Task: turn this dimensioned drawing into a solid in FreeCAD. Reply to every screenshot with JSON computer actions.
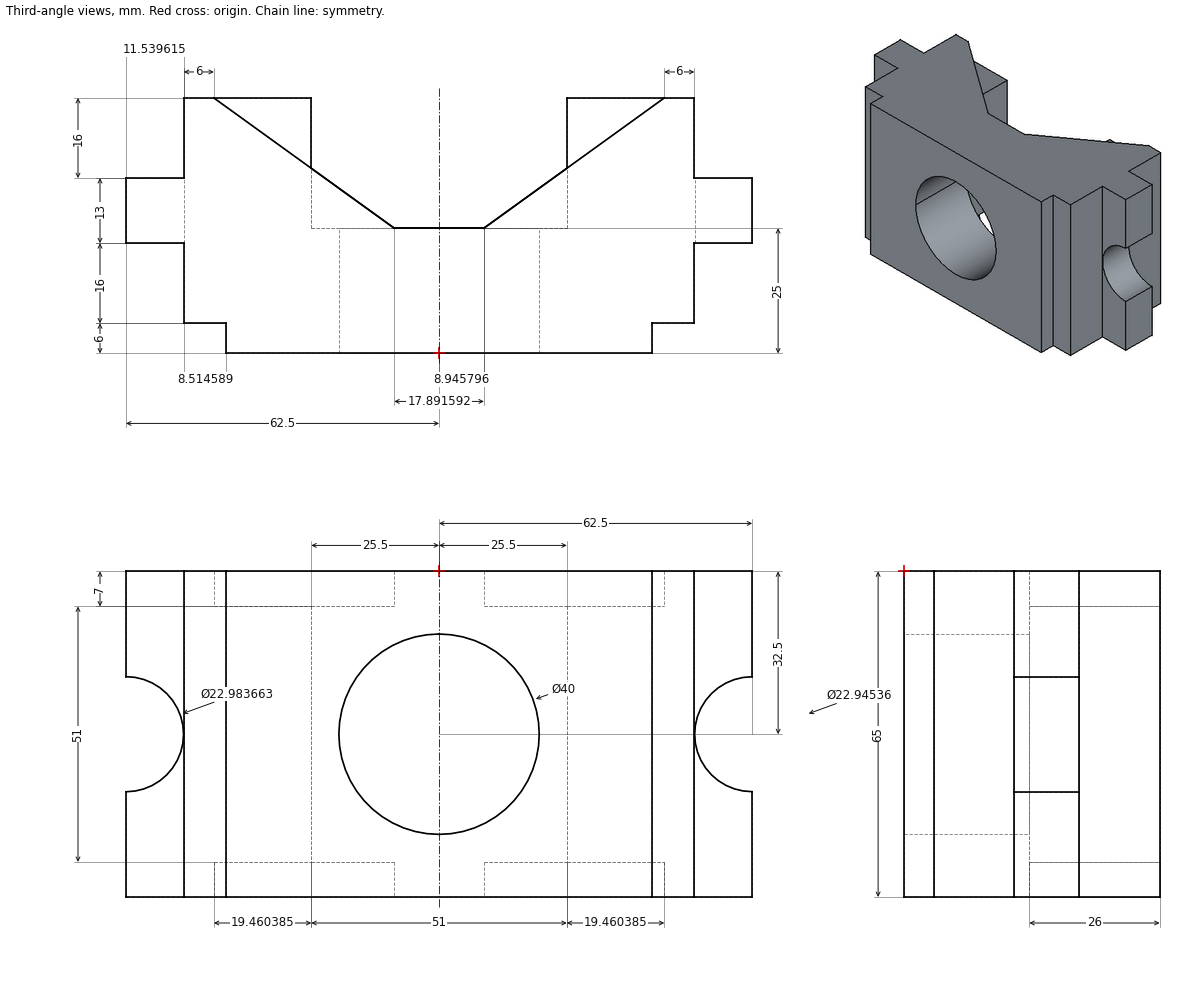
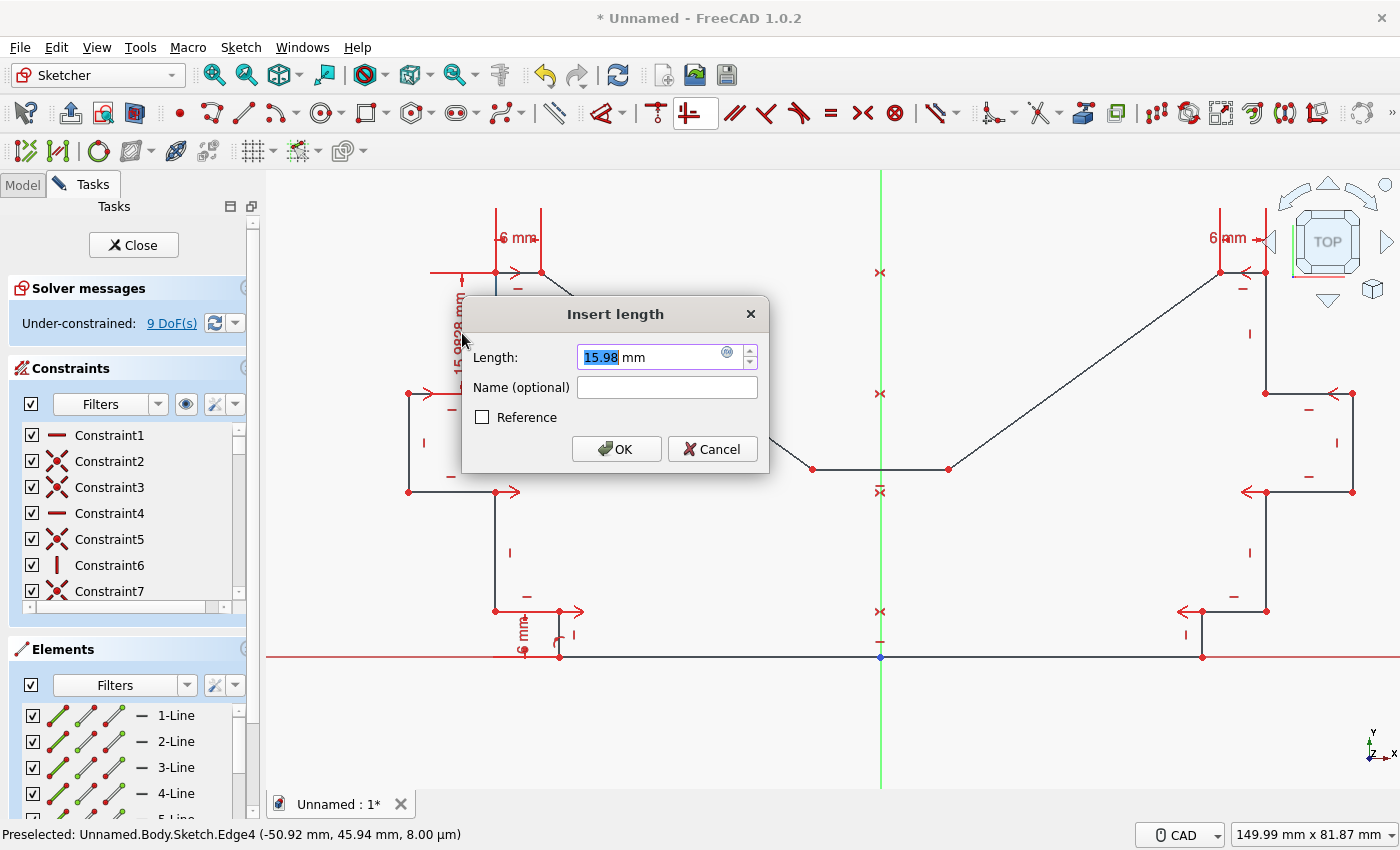
{"action": "type", "text": "16"}
{"action": "key", "text": "Return"}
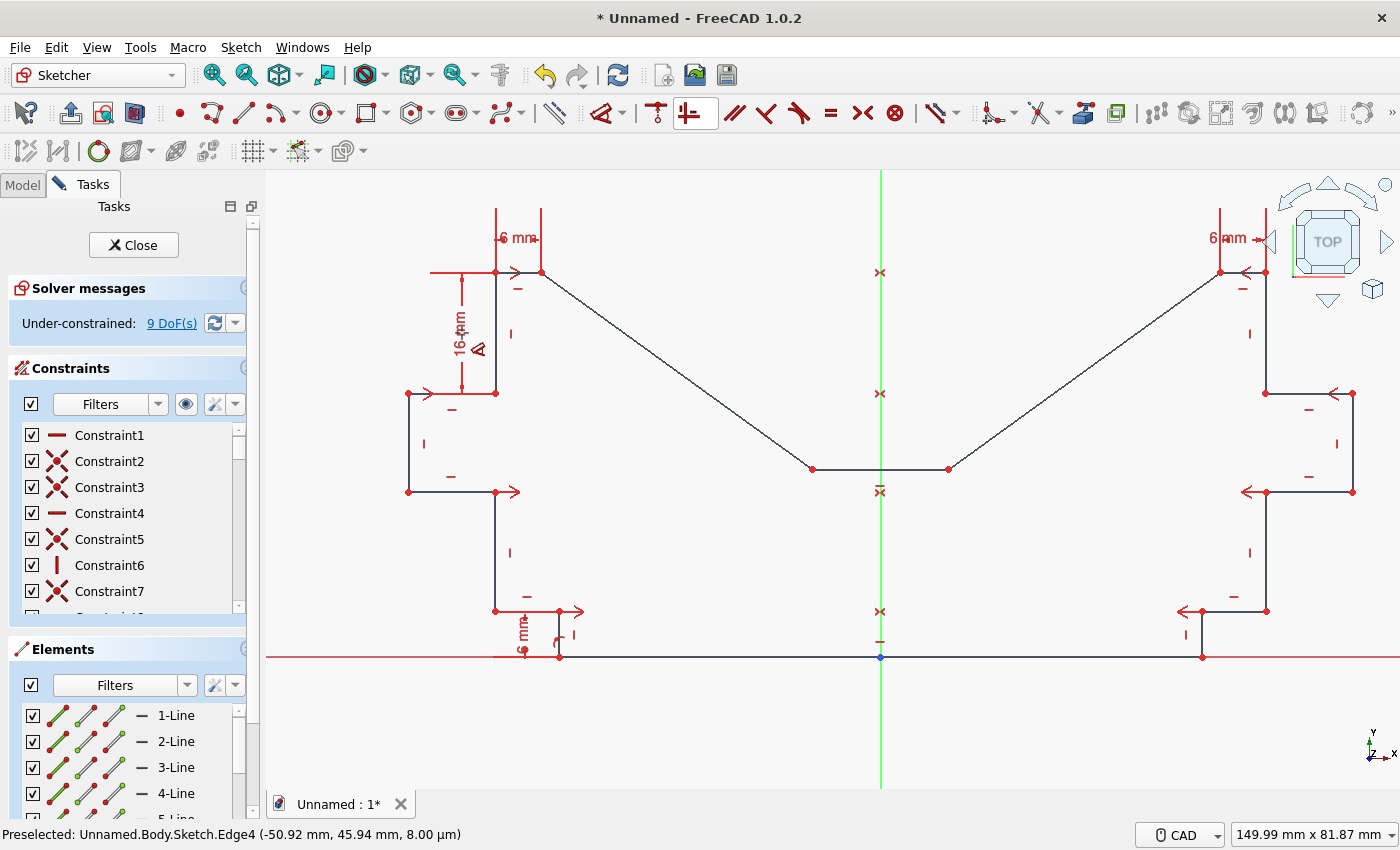
{"action": "left_click", "coordinate": [409, 423]}
{"action": "left_click", "coordinate": [375, 443]}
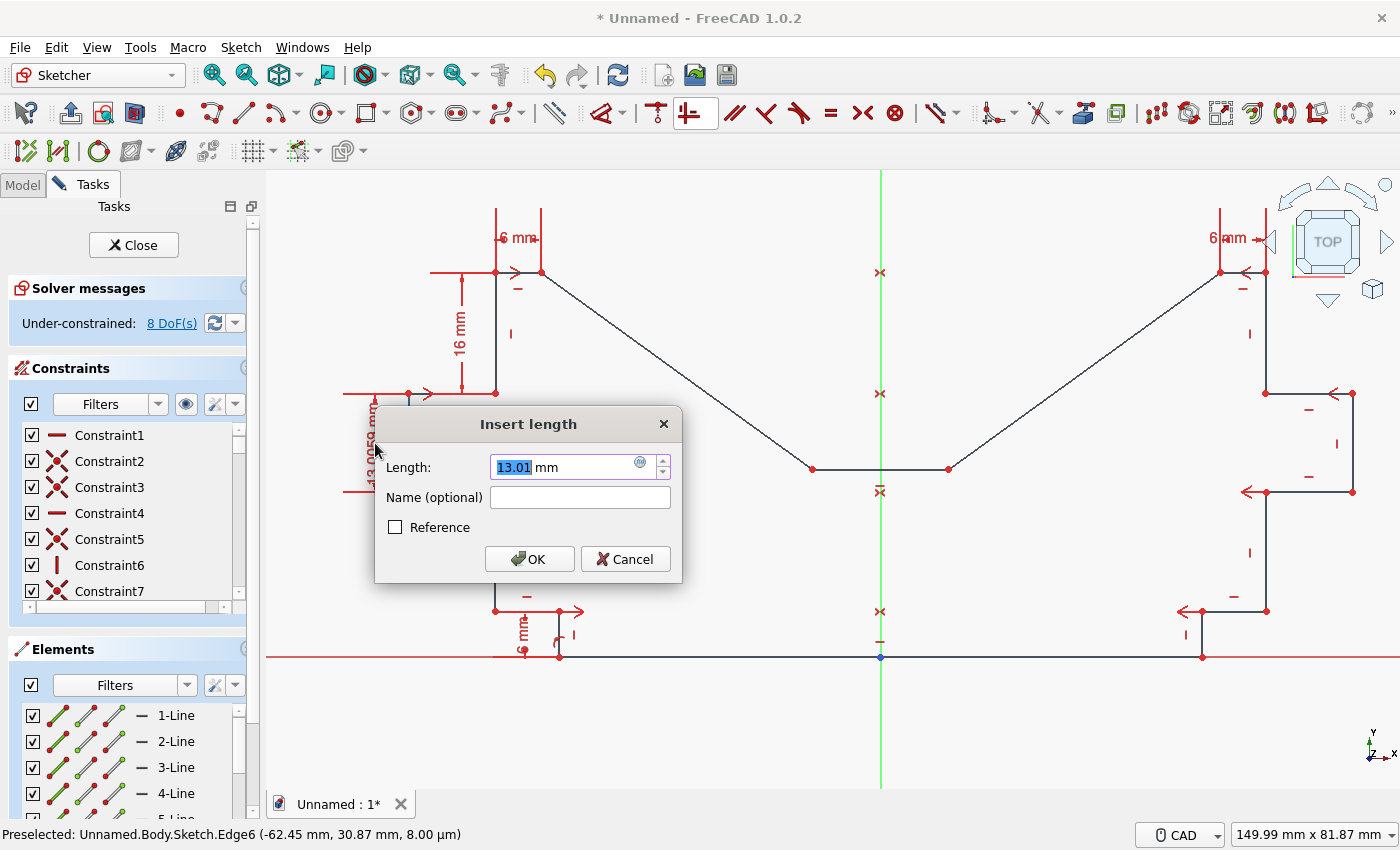
{"action": "type", "text": "13"}
{"action": "key", "text": "Return"}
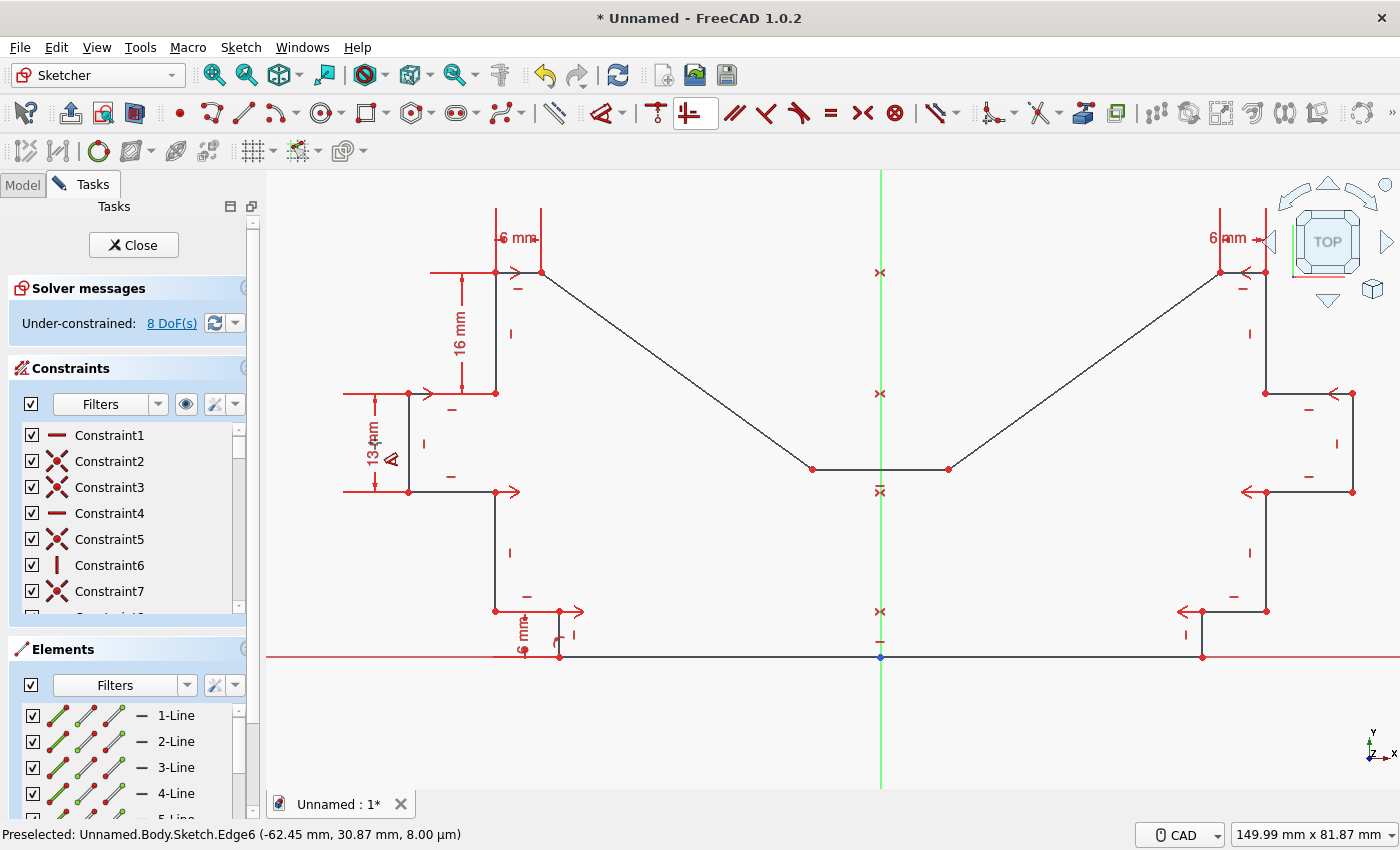
{"action": "left_click", "coordinate": [495, 528]}
{"action": "left_click", "coordinate": [461, 552]}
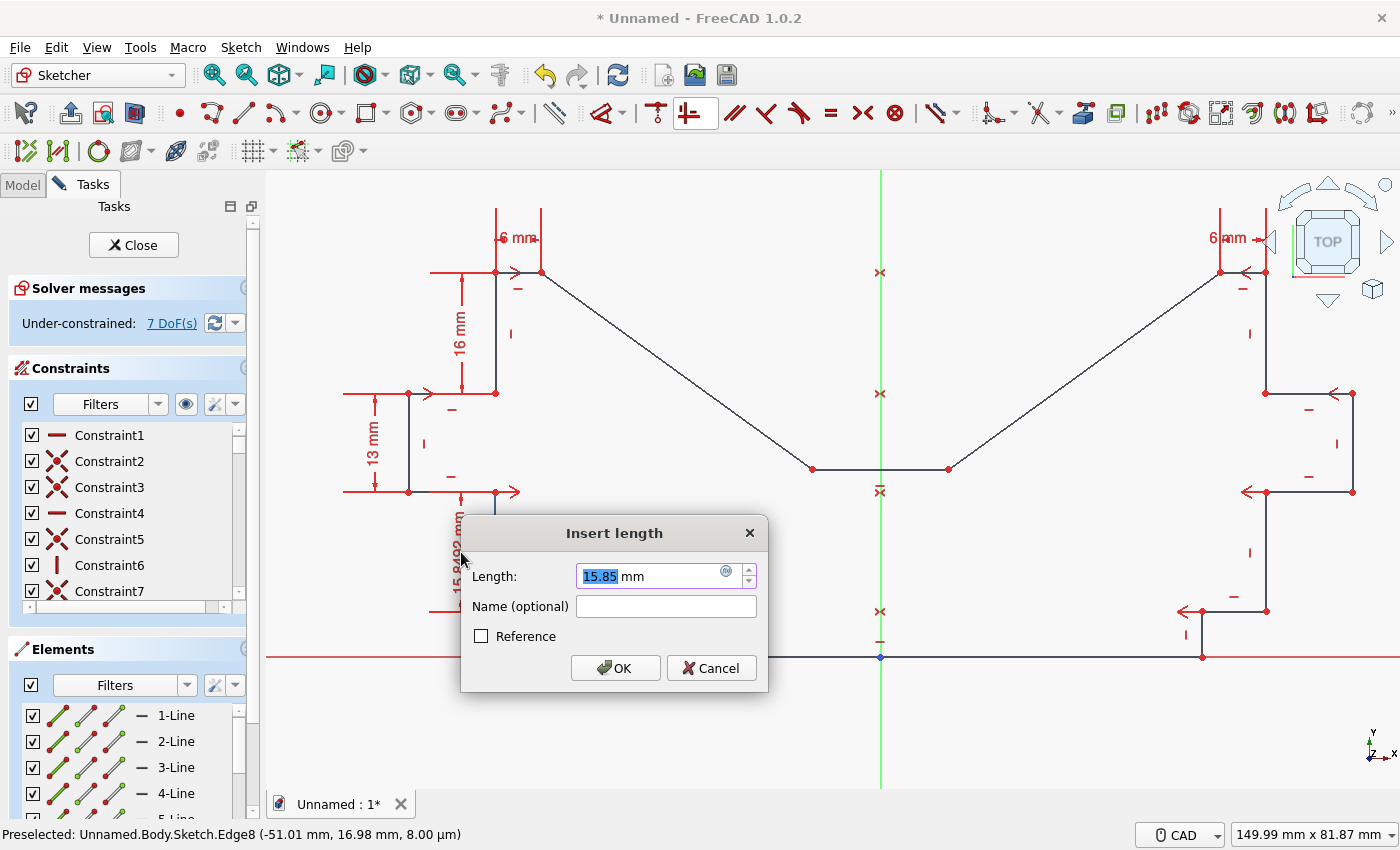
{"action": "type", "text": "16"}
{"action": "key", "text": "Return"}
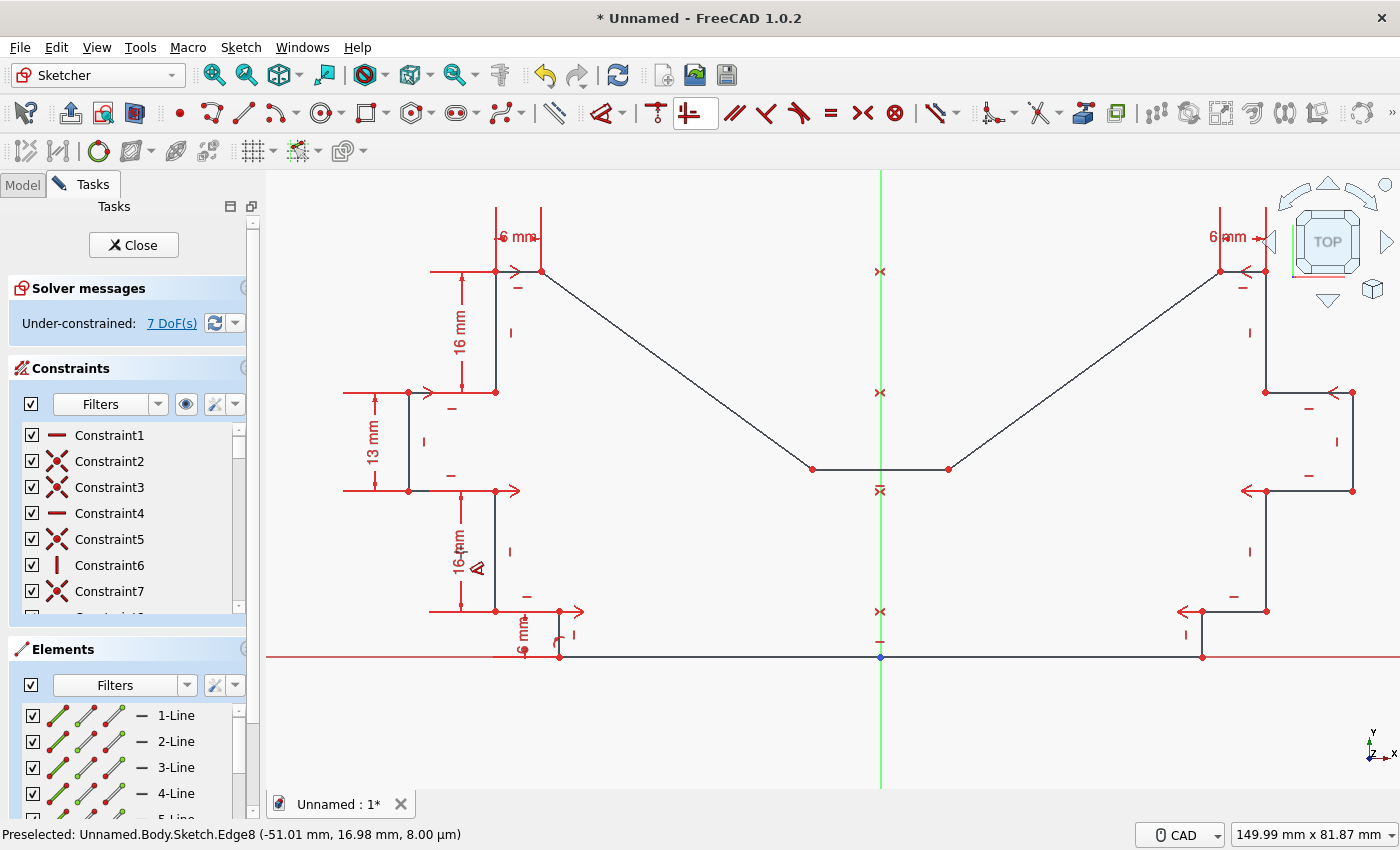
{"action": "left_click", "coordinate": [949, 470]}
{"action": "left_click", "coordinate": [983, 564]}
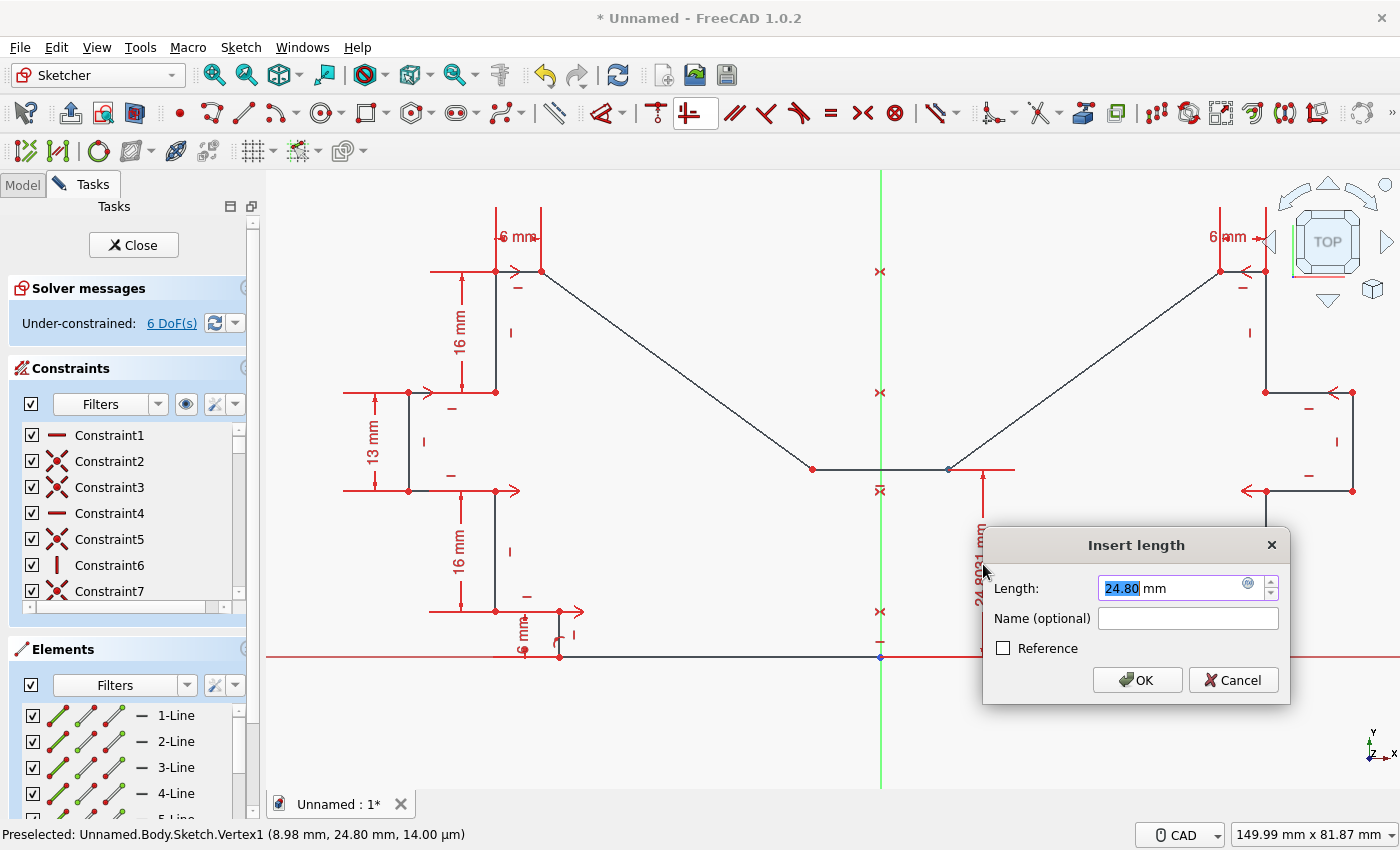
{"action": "type", "text": "25"}
{"action": "key", "text": "Return"}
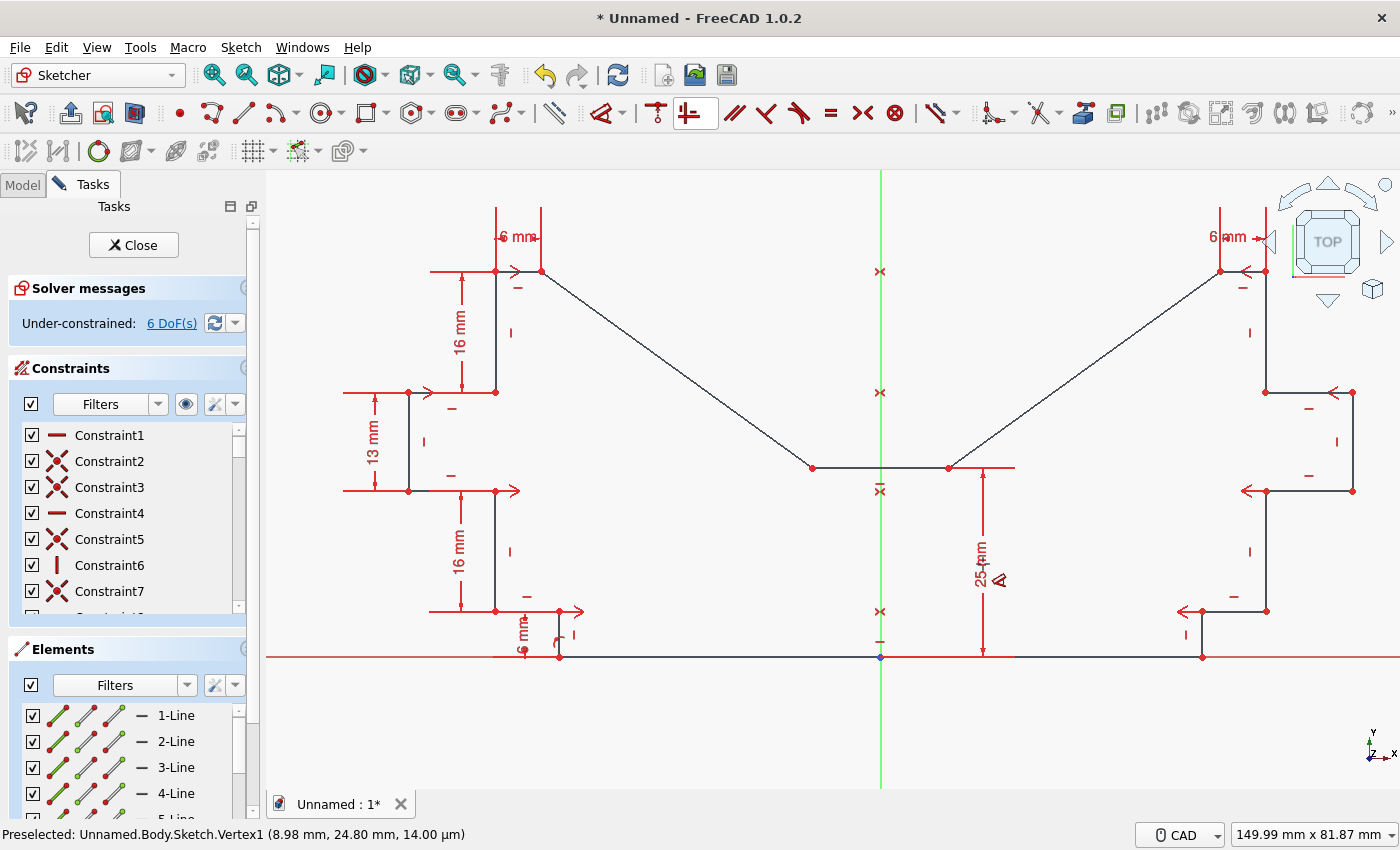
{"action": "left_click", "coordinate": [409, 393]}
{"action": "left_click", "coordinate": [645, 691]}